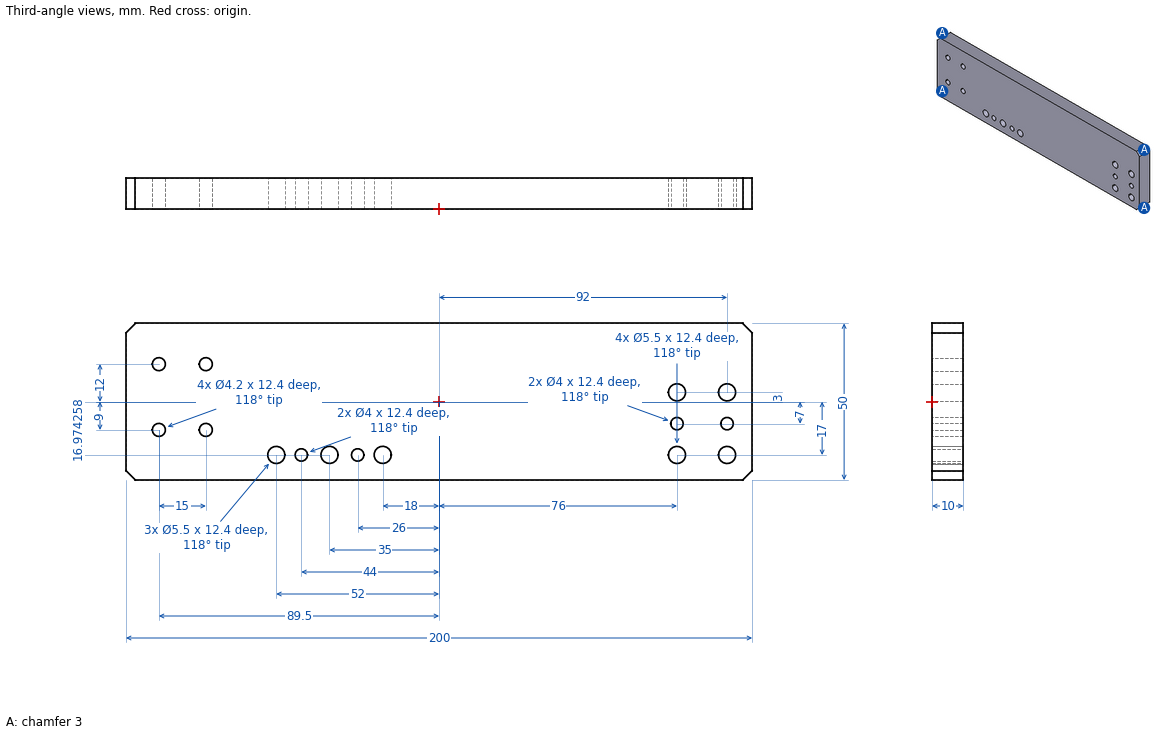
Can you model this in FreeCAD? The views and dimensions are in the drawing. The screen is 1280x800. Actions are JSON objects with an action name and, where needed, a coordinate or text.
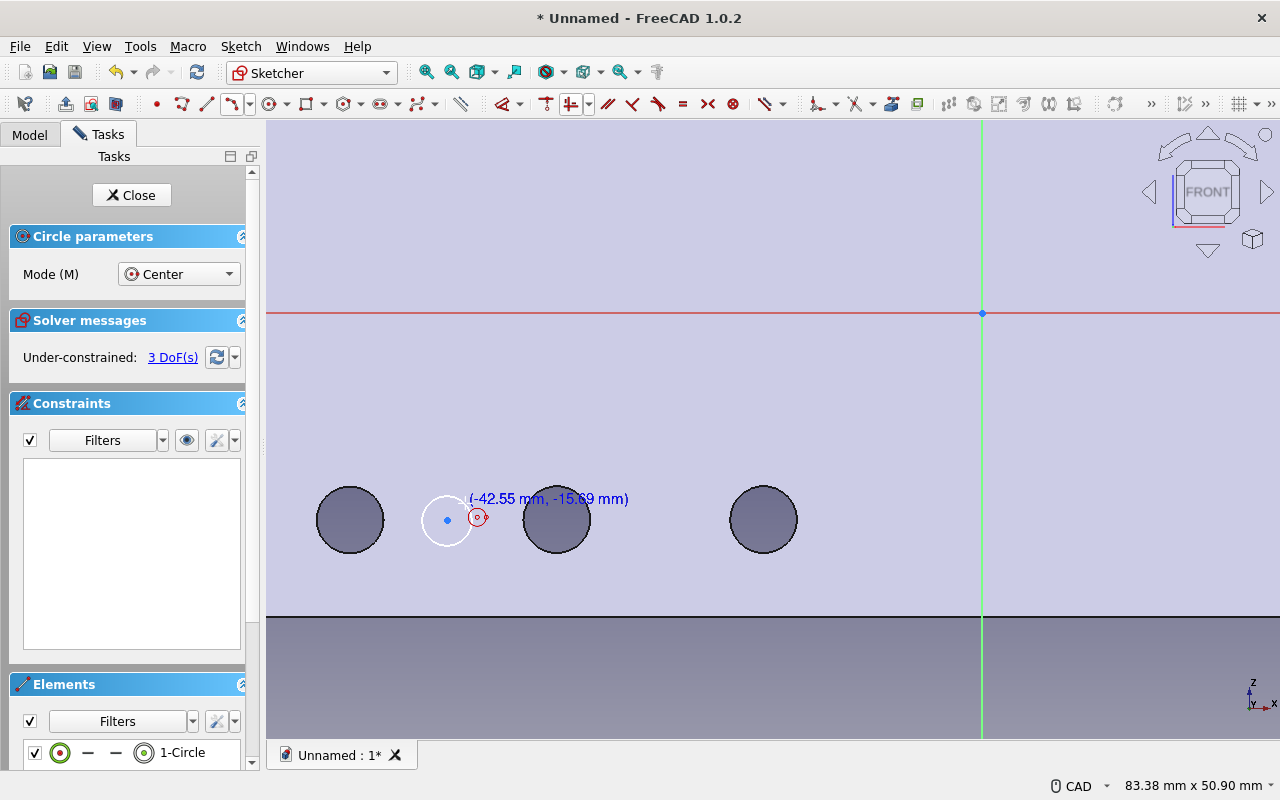
{"action": "left_click", "coordinate": [666, 520]}
{"action": "left_click", "coordinate": [683, 503]}
{"action": "key", "text": "Escape"}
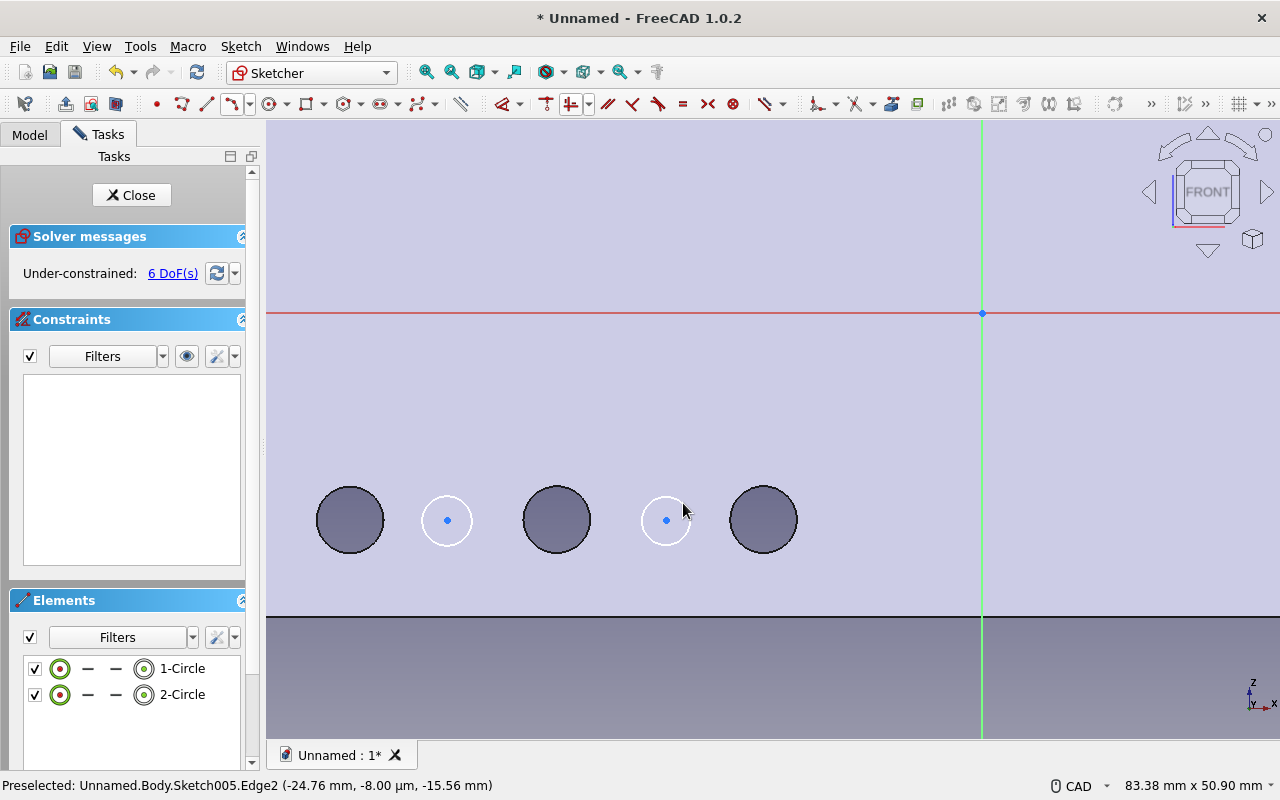
{"action": "left_click", "coordinate": [464, 503]}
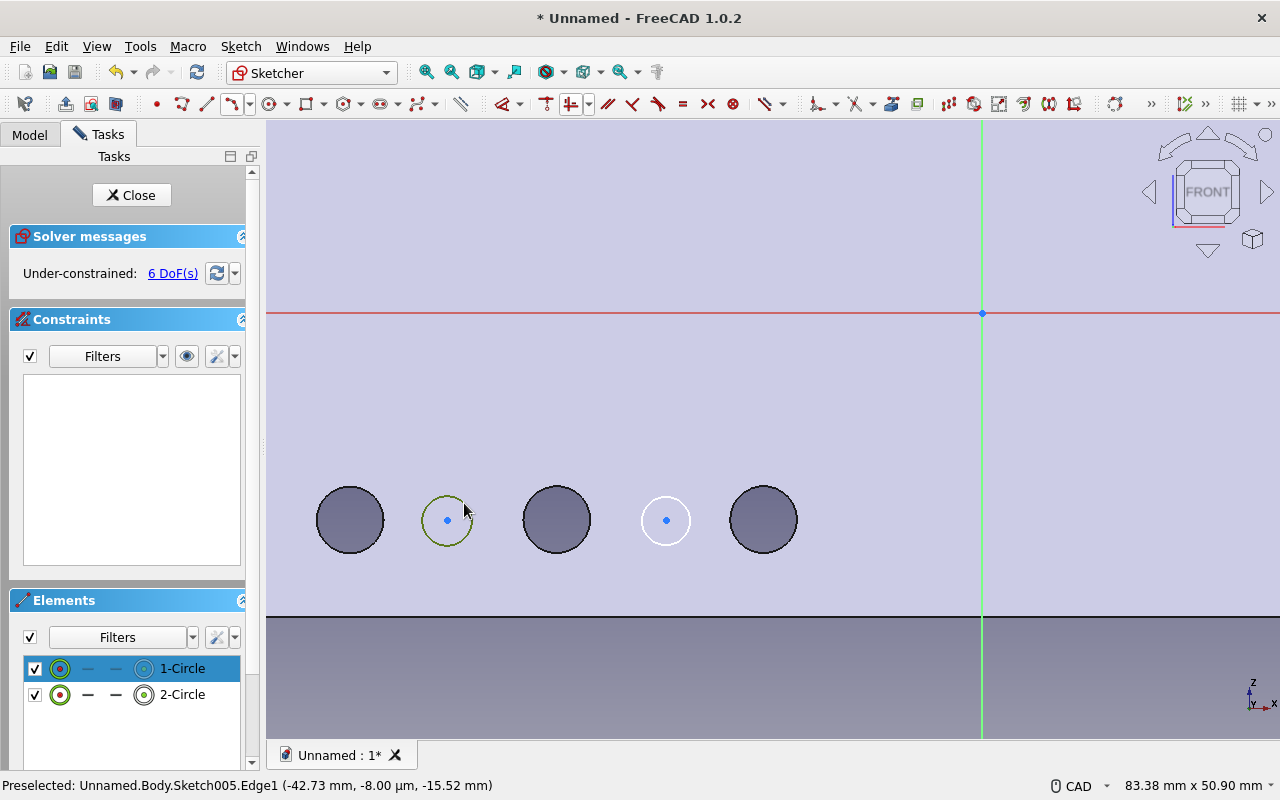
{"action": "left_click", "coordinate": [683, 504]}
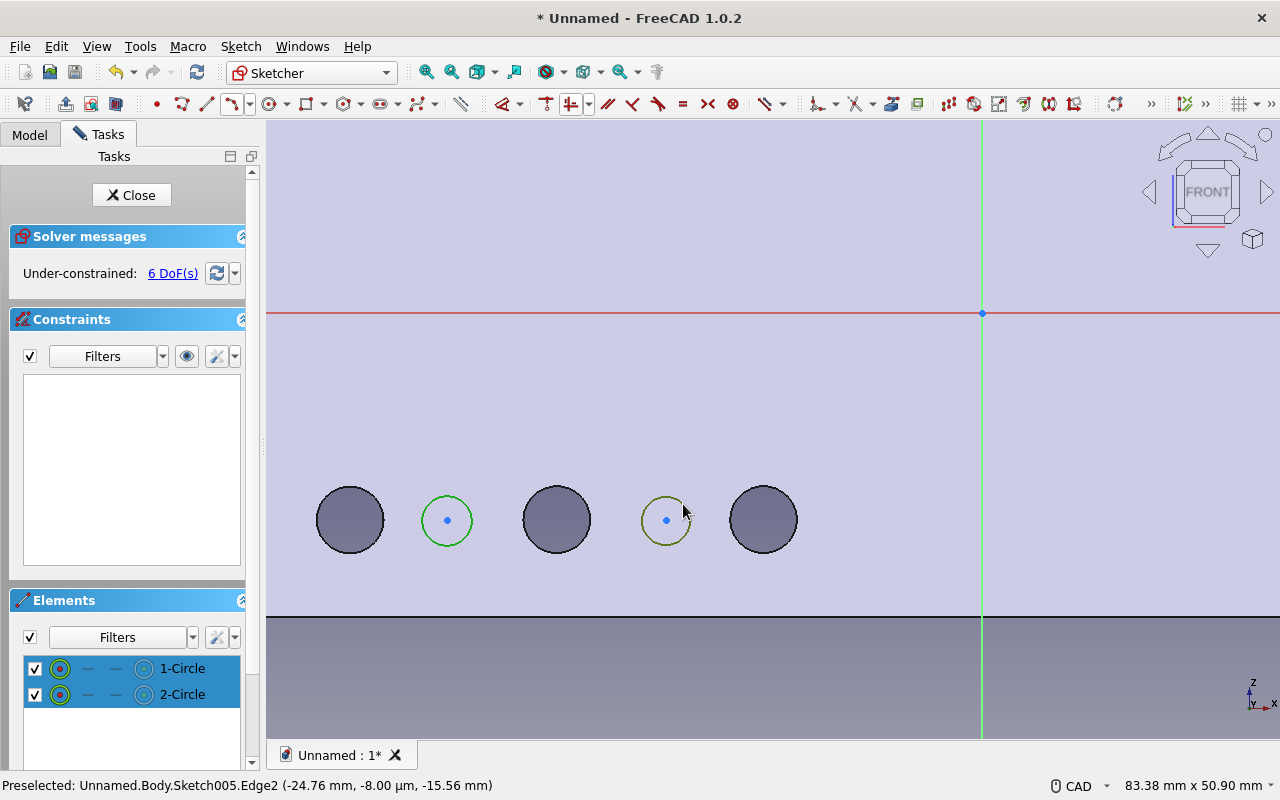
{"action": "key", "text": "e"}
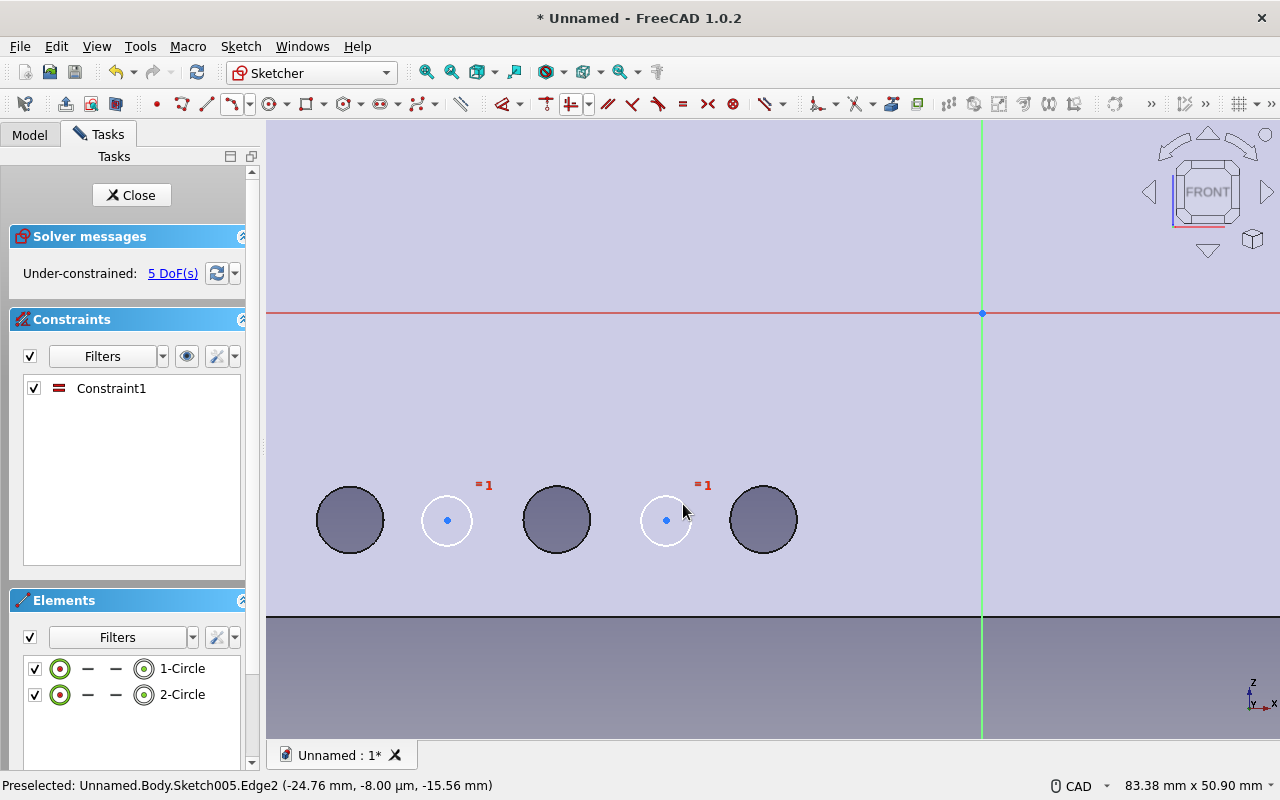
{"action": "left_click", "coordinate": [447, 521]}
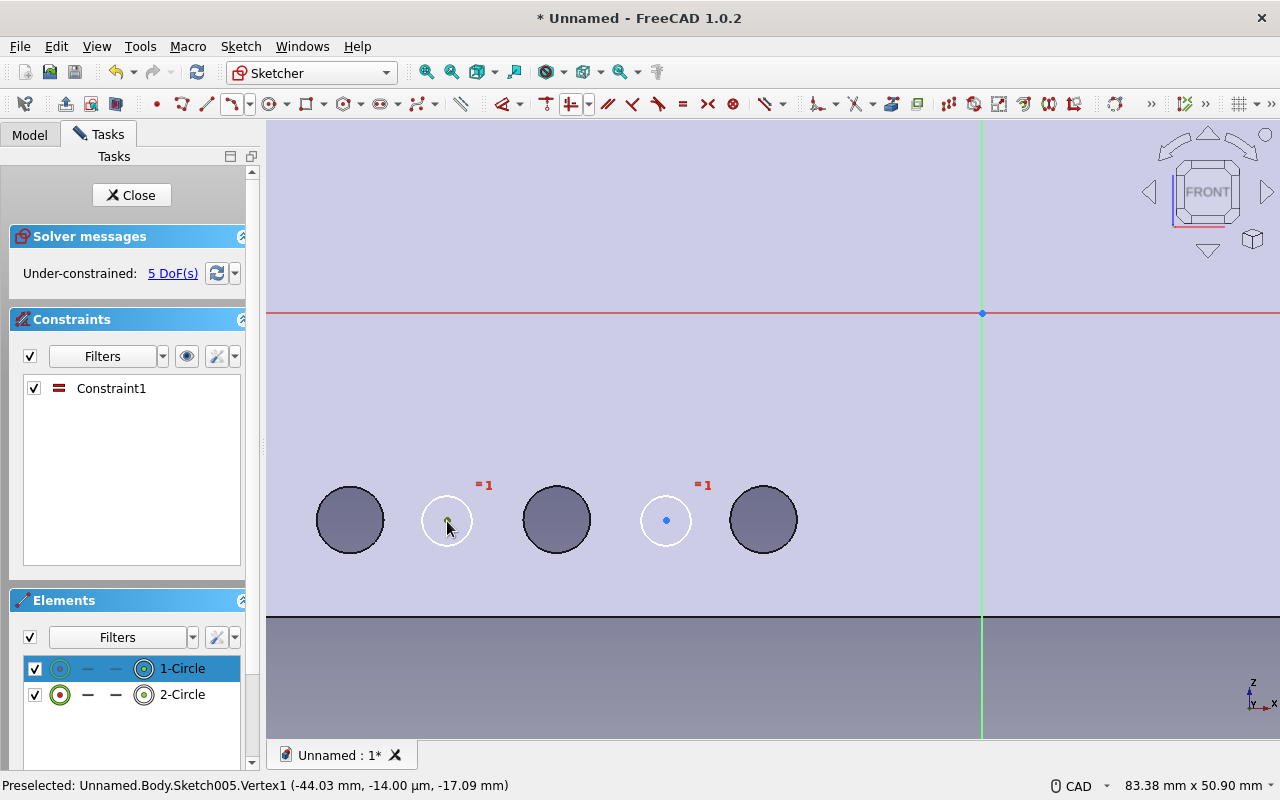
{"action": "left_click", "coordinate": [666, 521]}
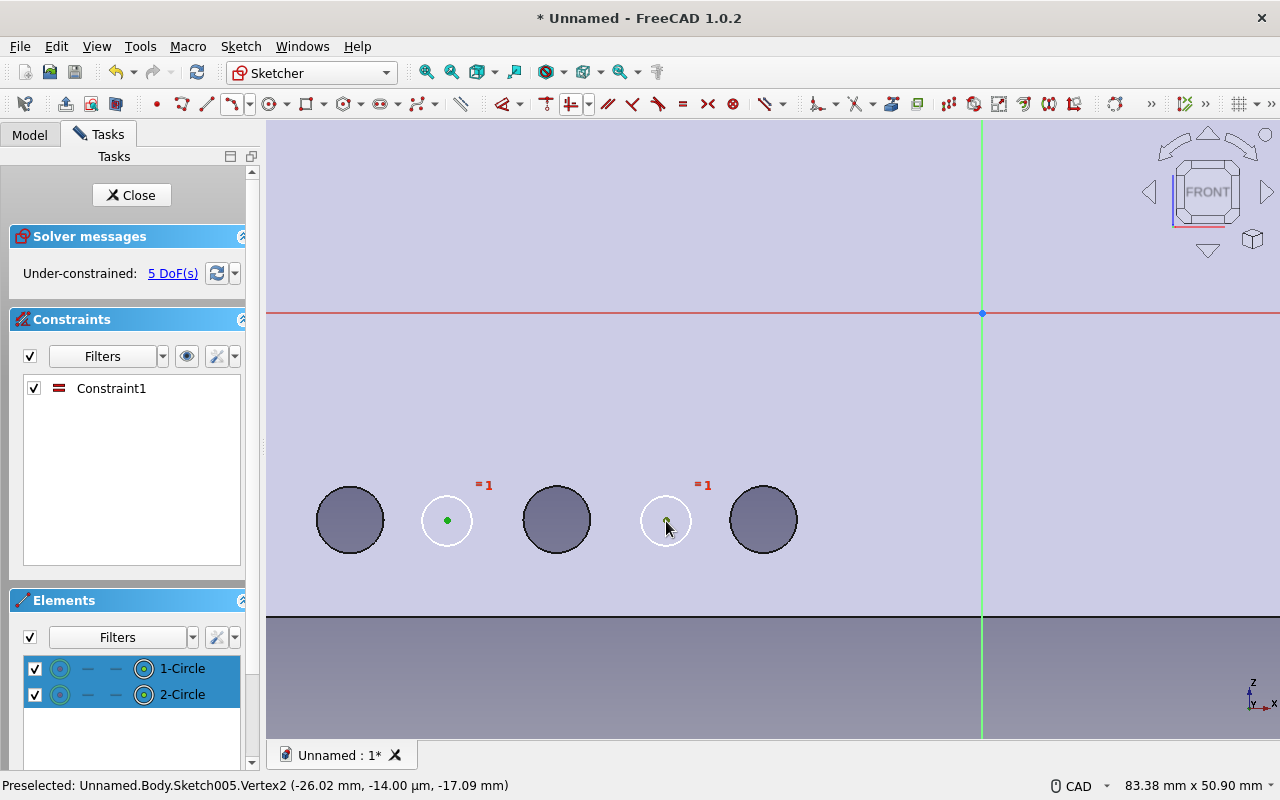
{"action": "left_click", "coordinate": [588, 104]}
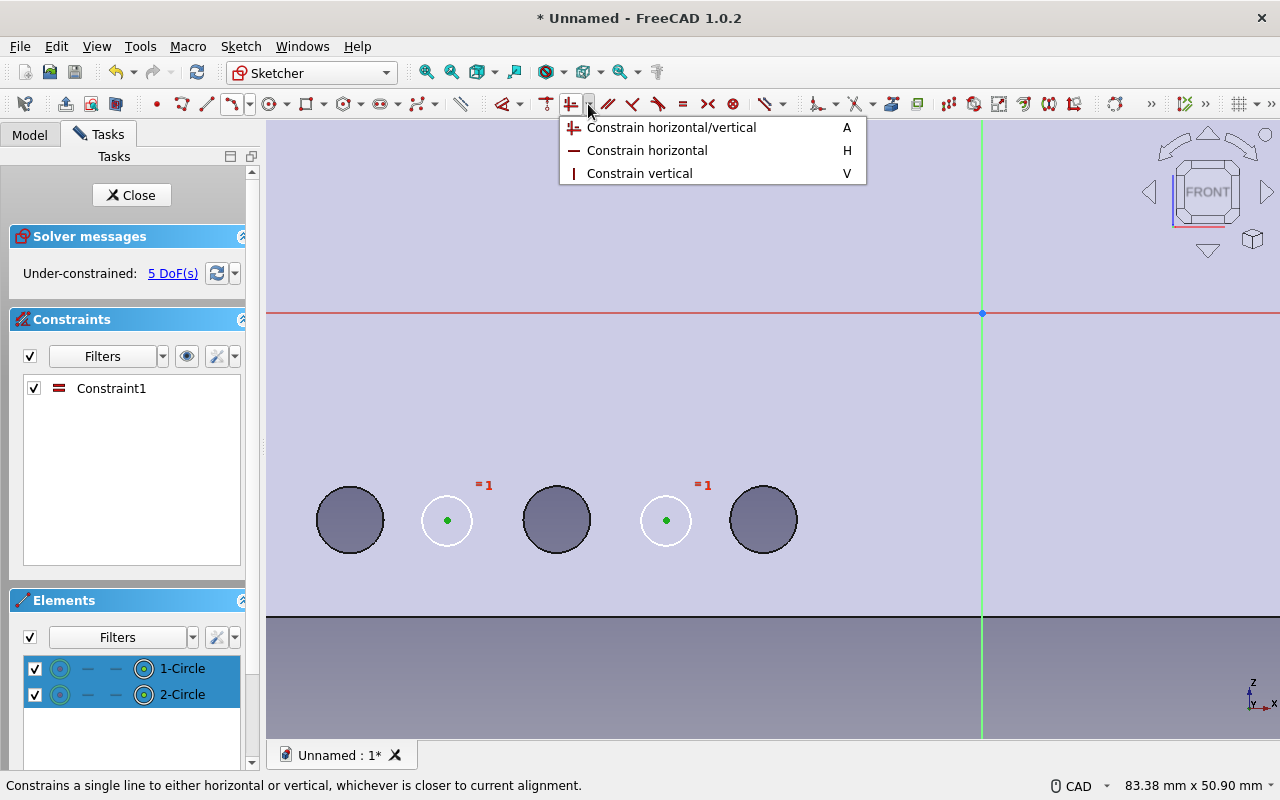
{"action": "left_click", "coordinate": [713, 150]}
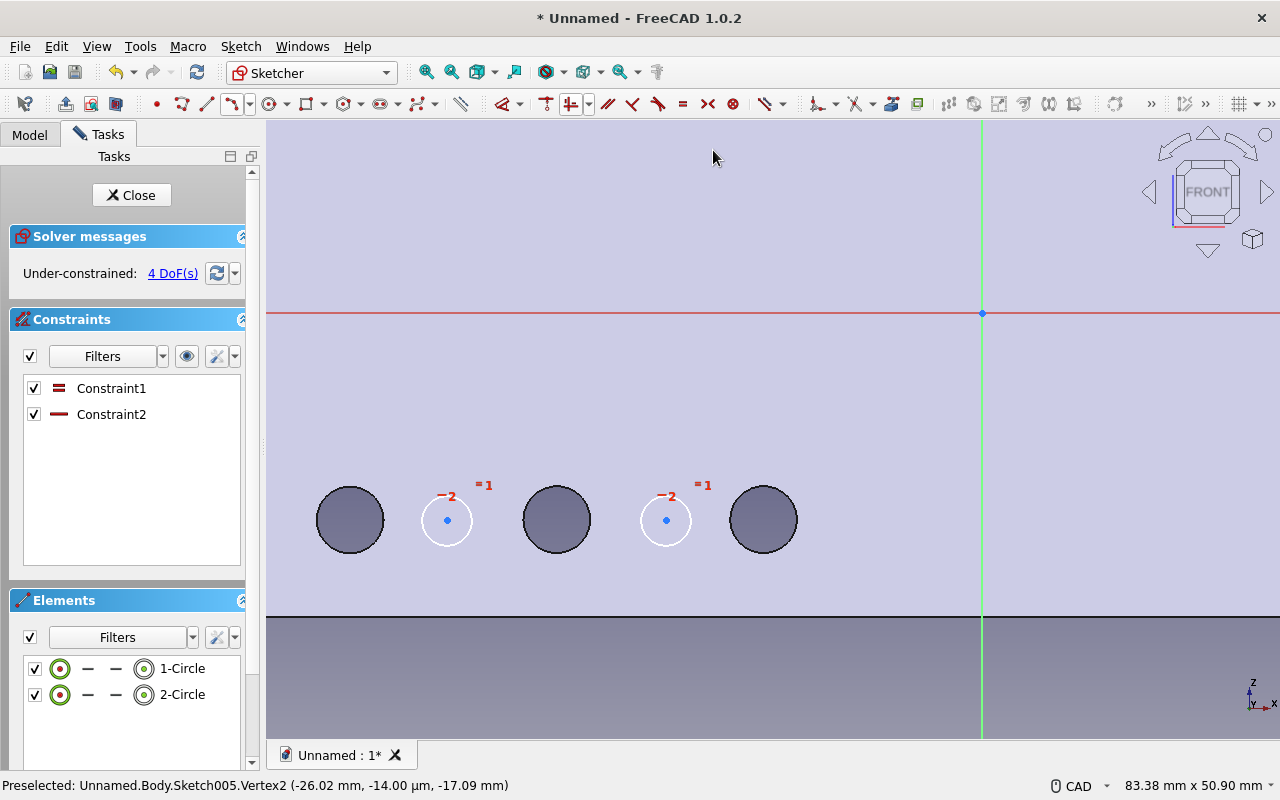
{"action": "key", "text": "d"}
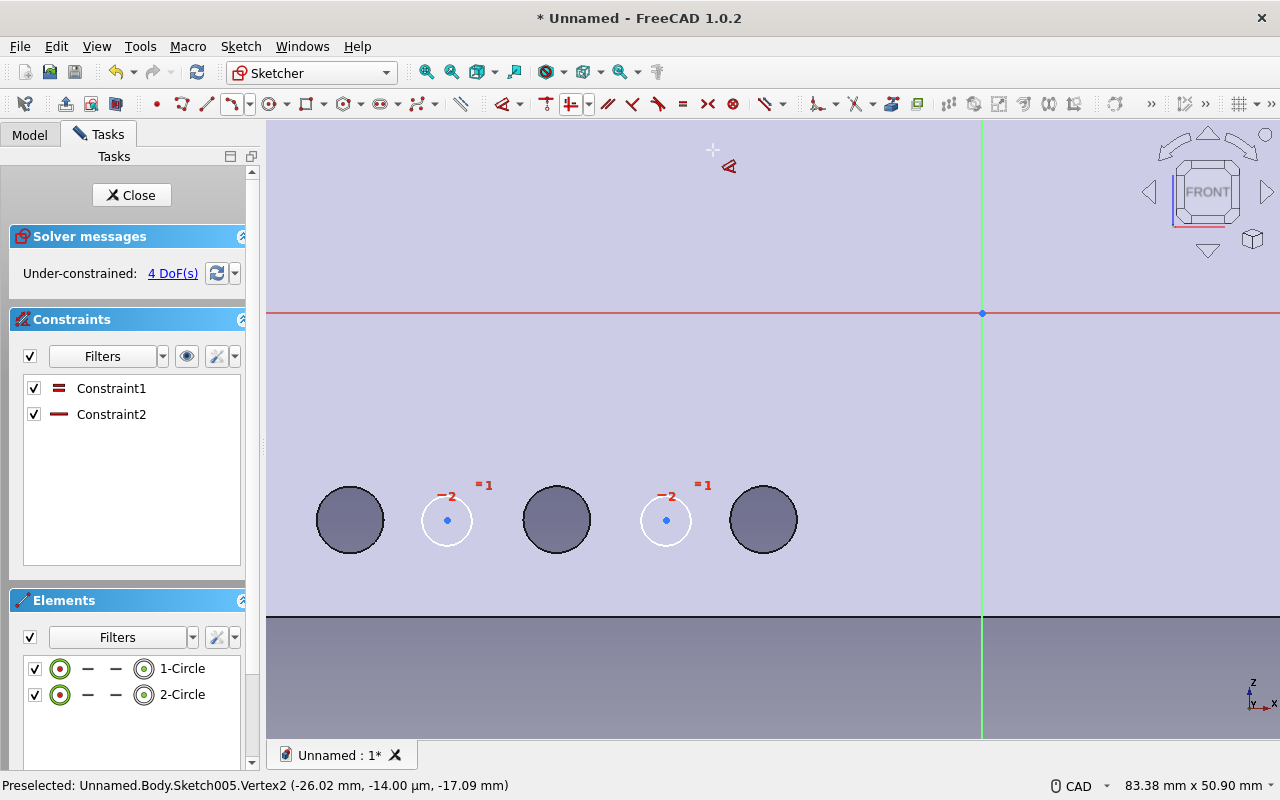
{"action": "left_click", "coordinate": [464, 503]}
{"action": "left_click", "coordinate": [486, 480]}